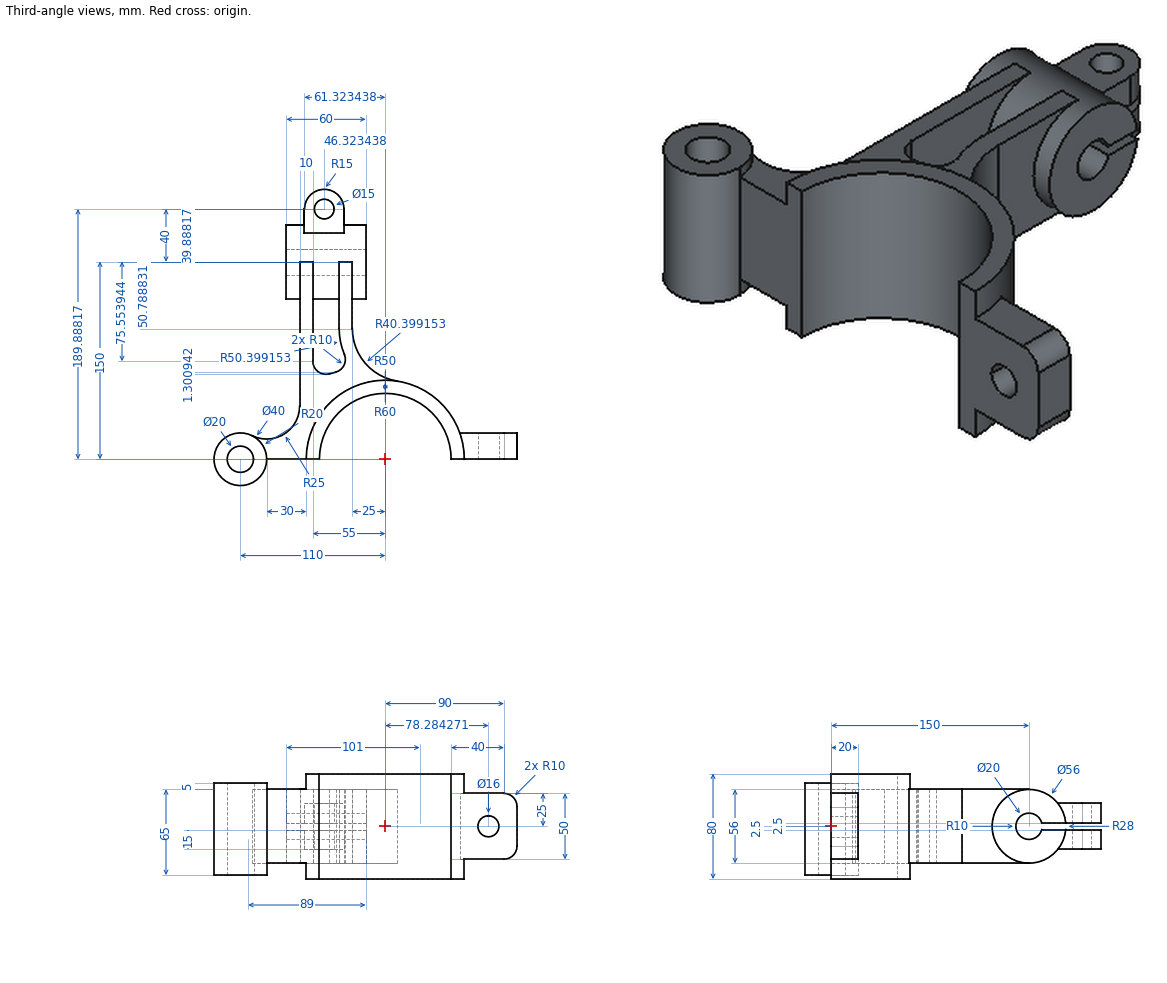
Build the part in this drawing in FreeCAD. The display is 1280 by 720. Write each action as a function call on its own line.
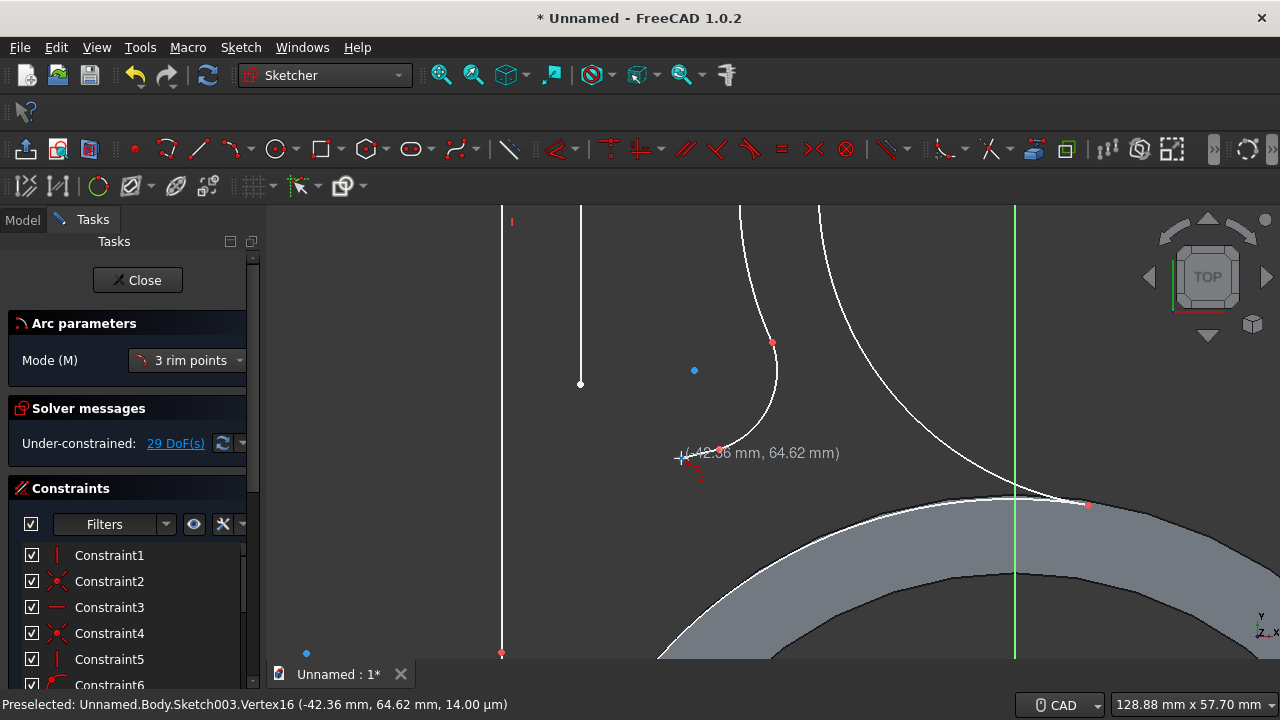
scroll(721, 450, down, 7)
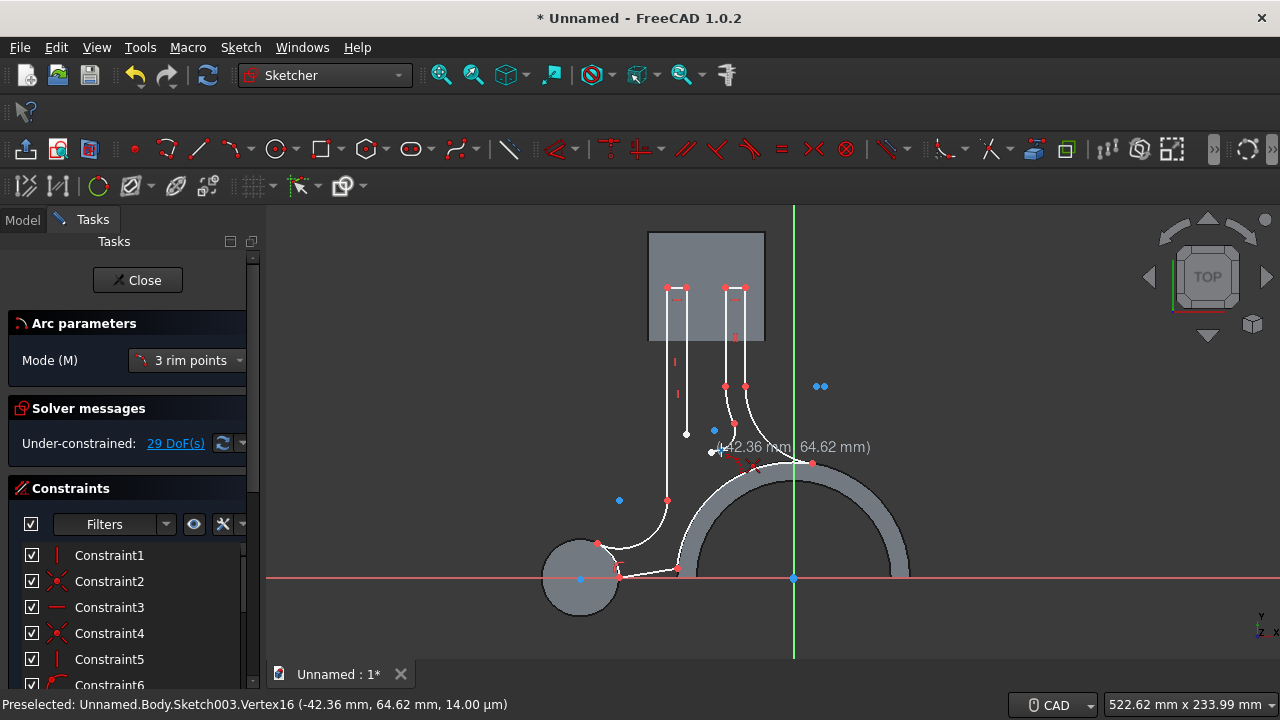
click(687, 434)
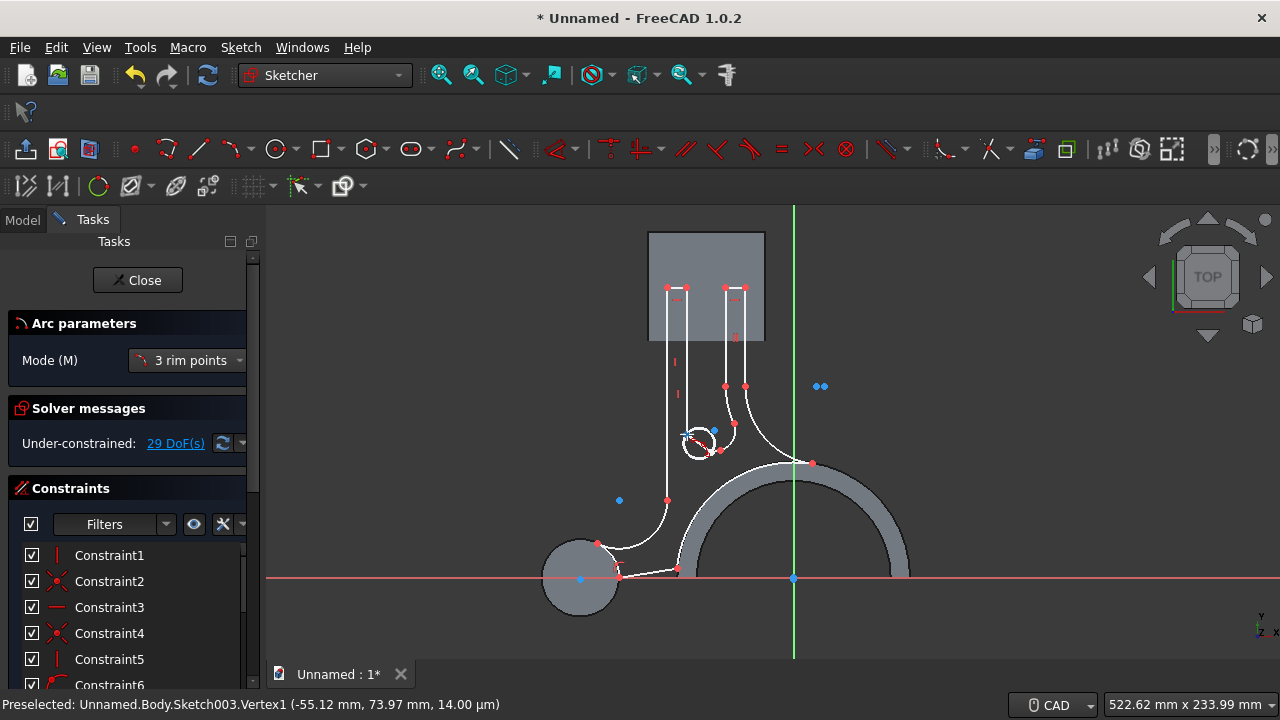
scroll(695, 449, up, 4)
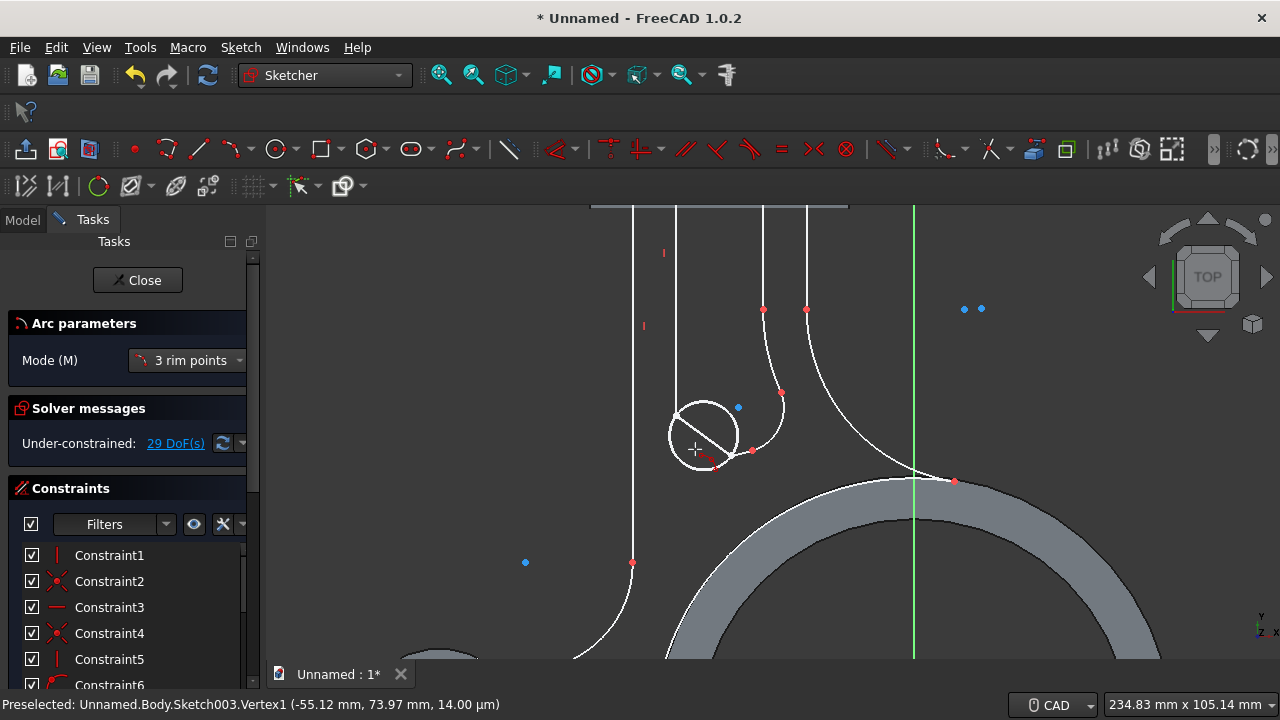
click(694, 448)
key(Escape)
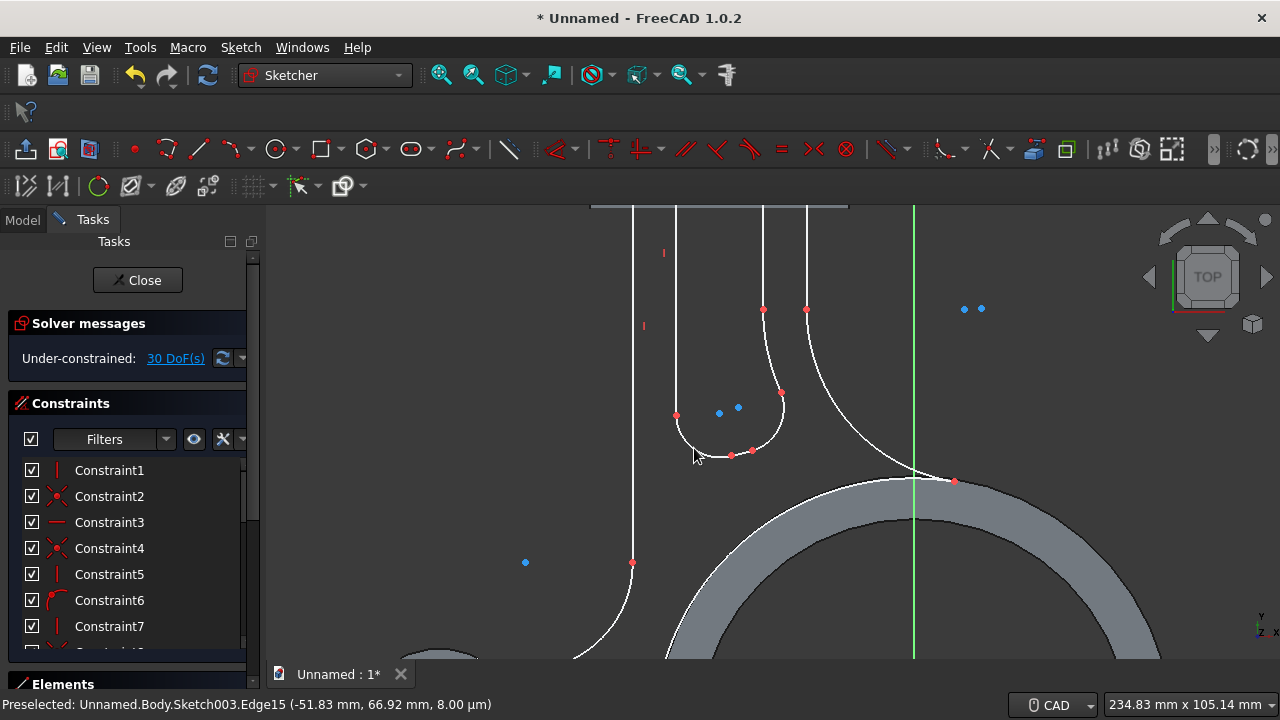
click(676, 318)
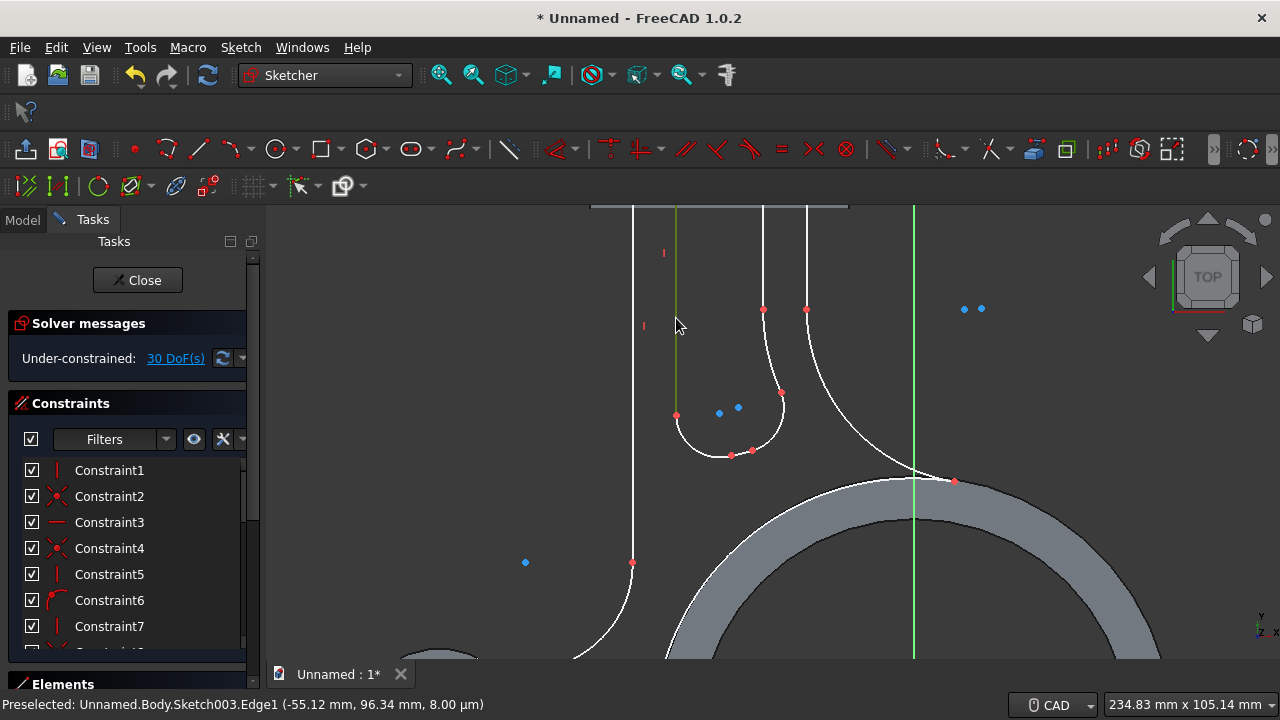
click(683, 438)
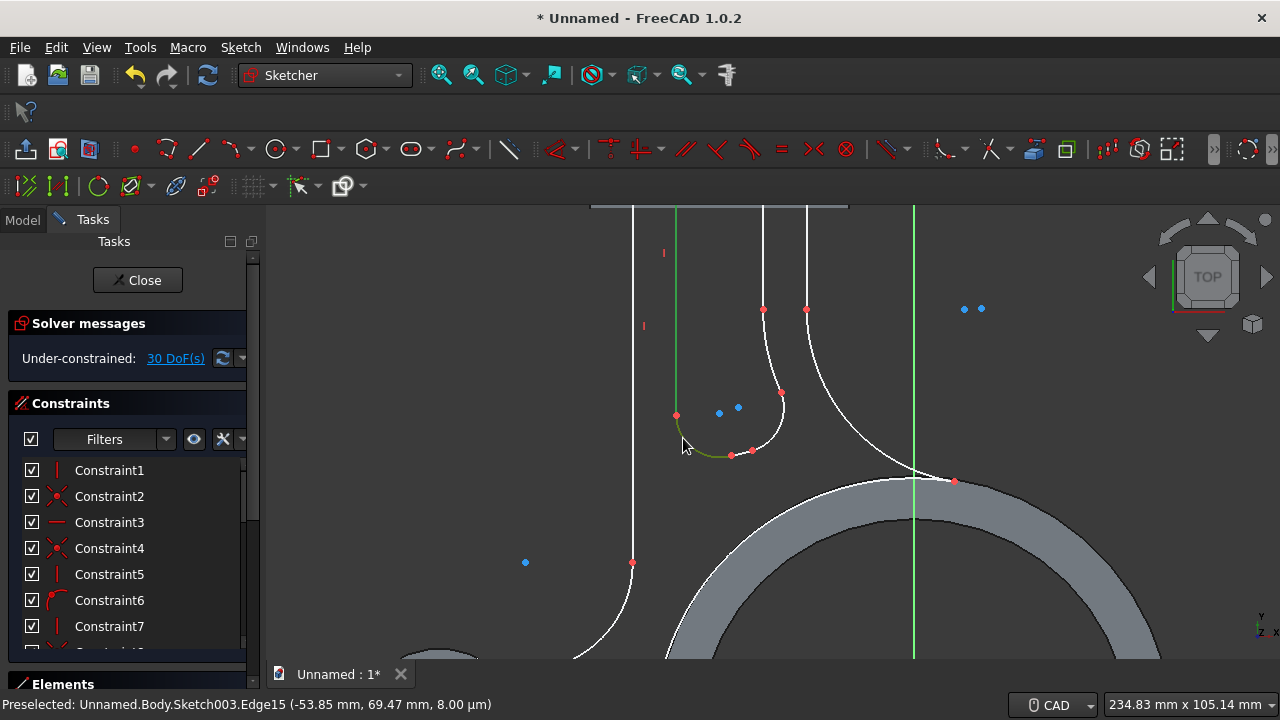
click(750, 150)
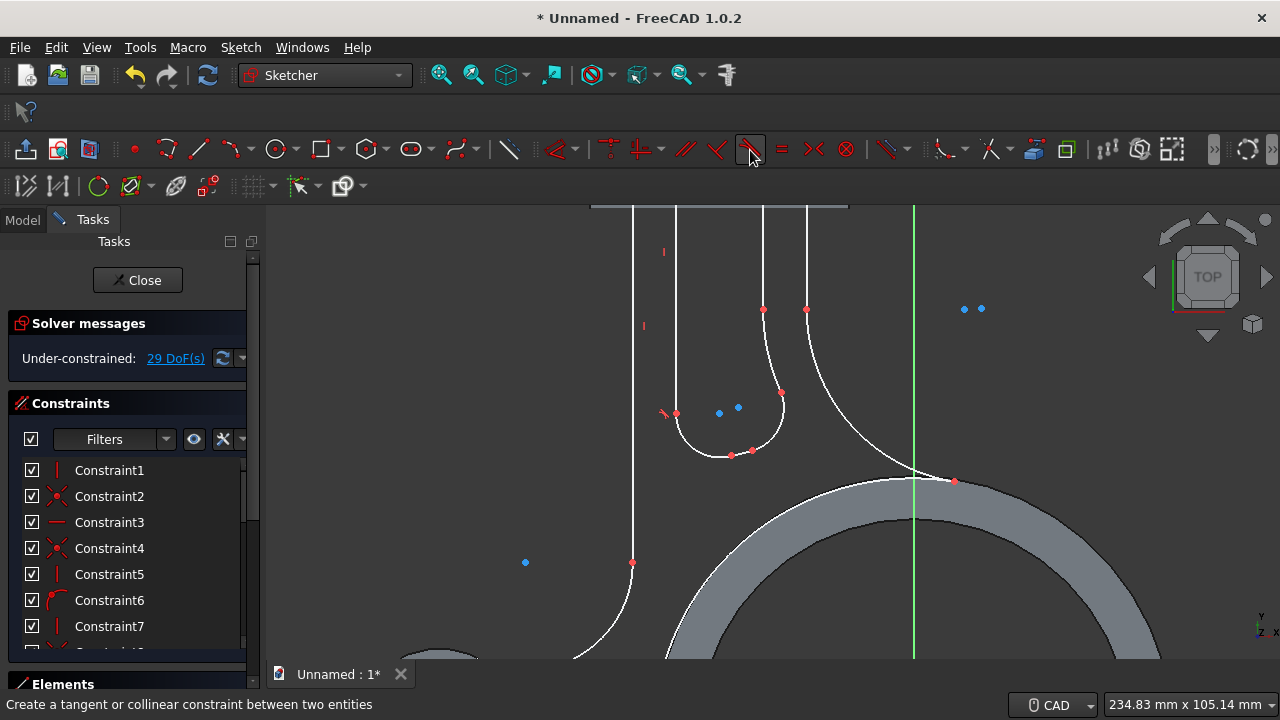
click(633, 421)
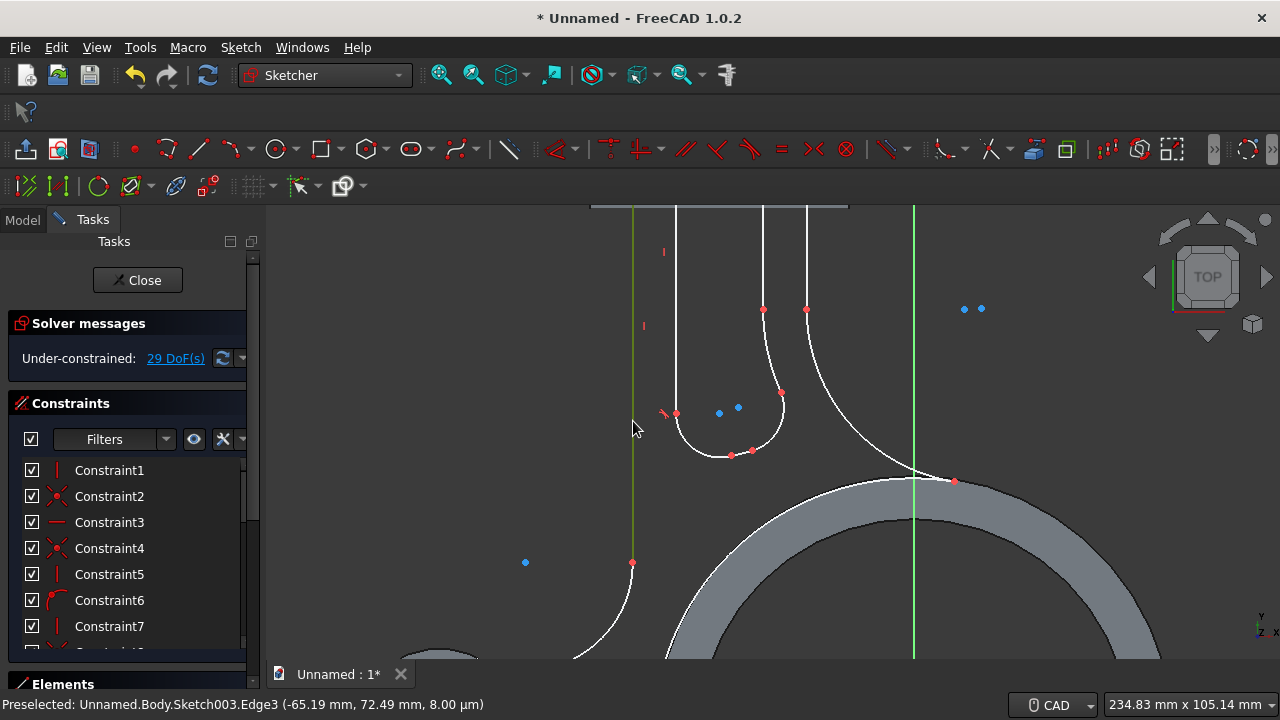
click(613, 624)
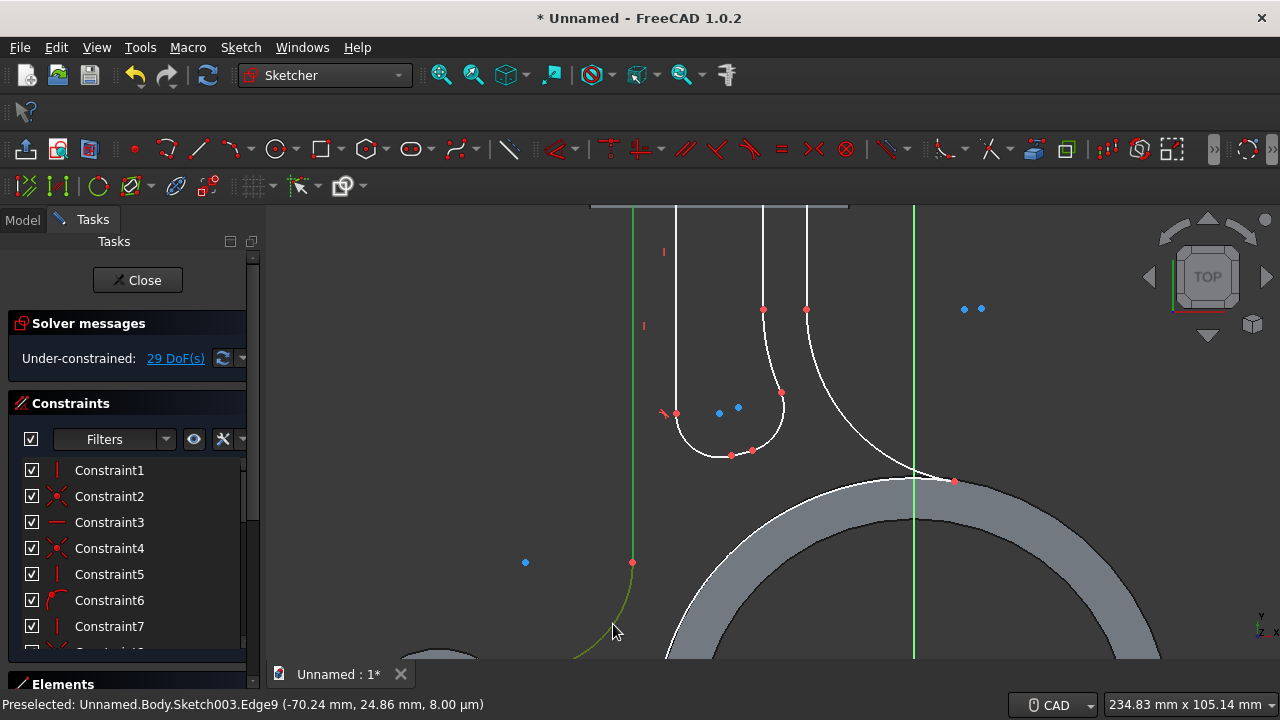
key(t)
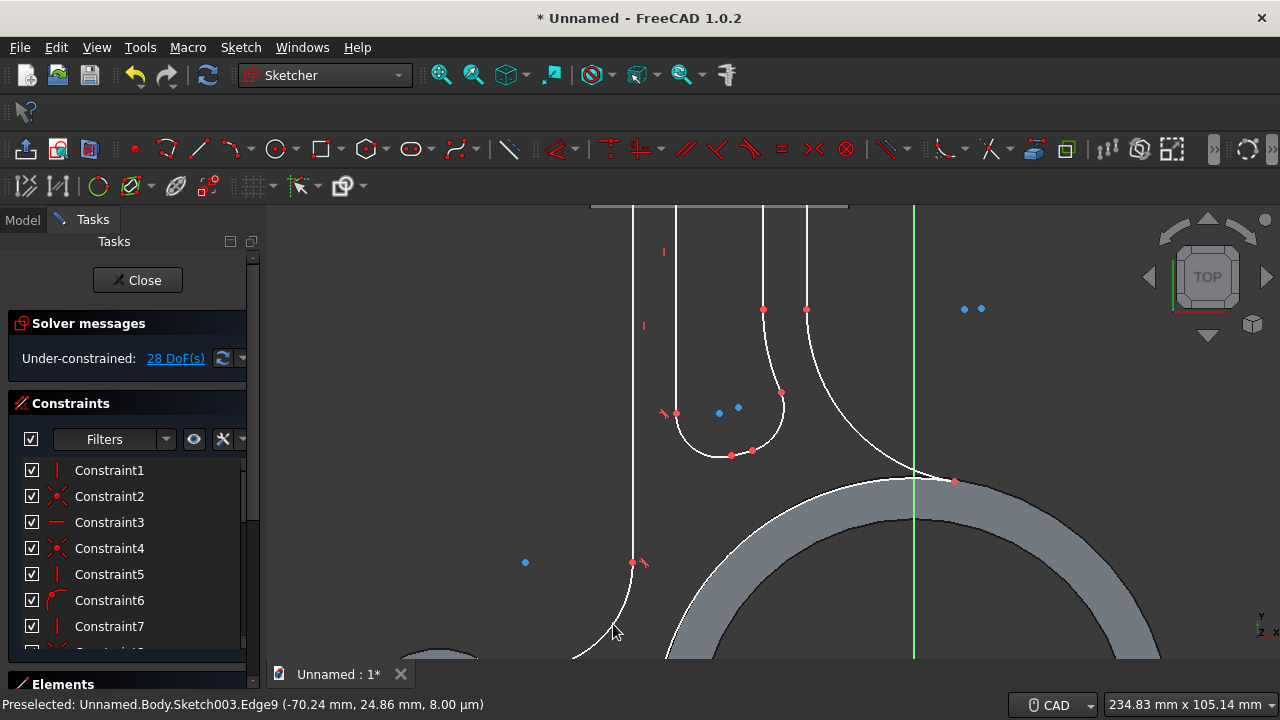
scroll(742, 453, up, 2)